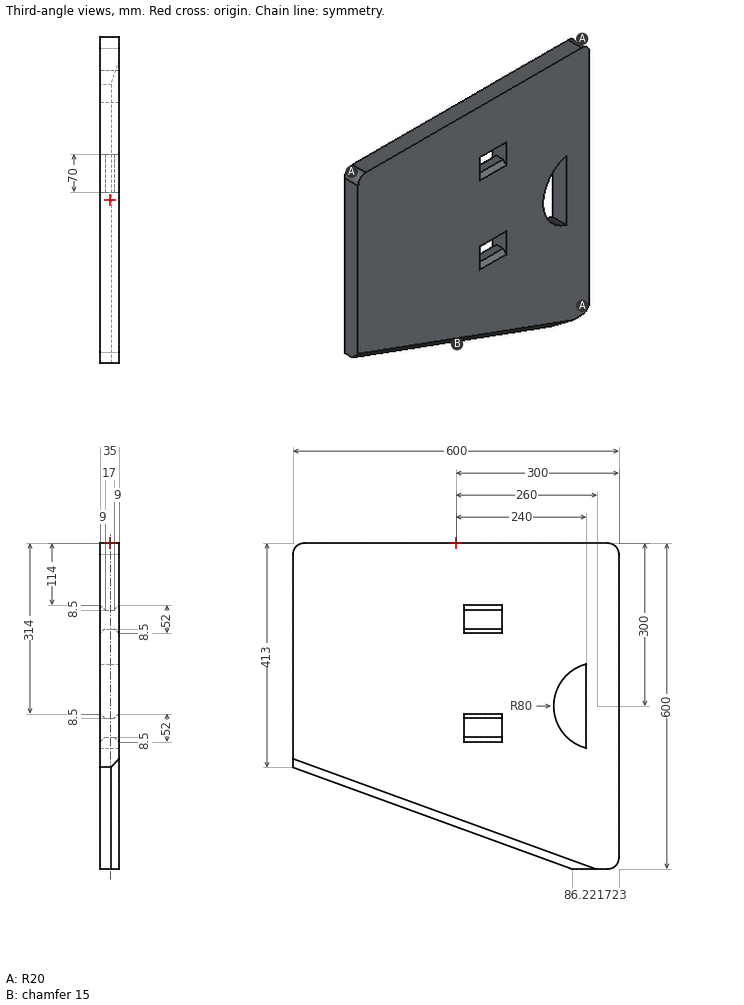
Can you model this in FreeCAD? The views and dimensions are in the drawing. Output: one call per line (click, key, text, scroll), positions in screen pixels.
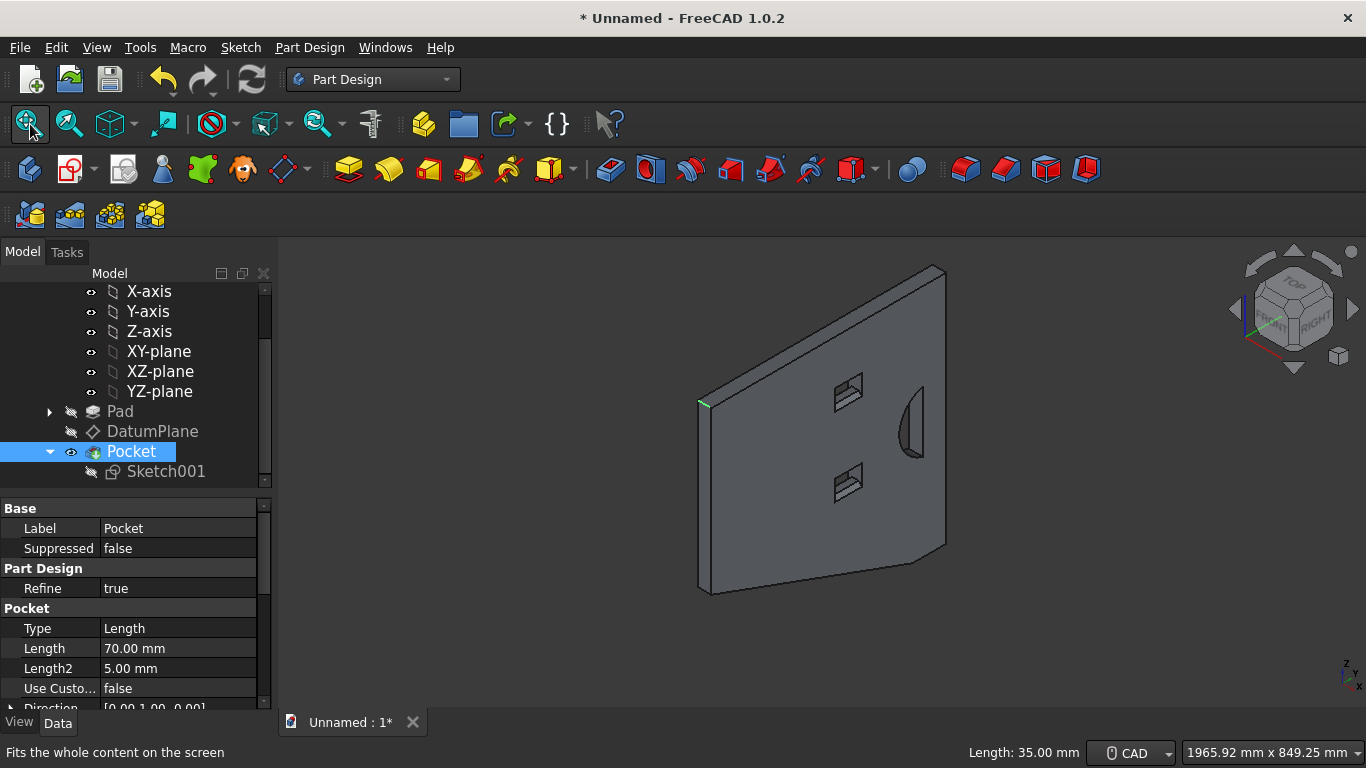
key(2)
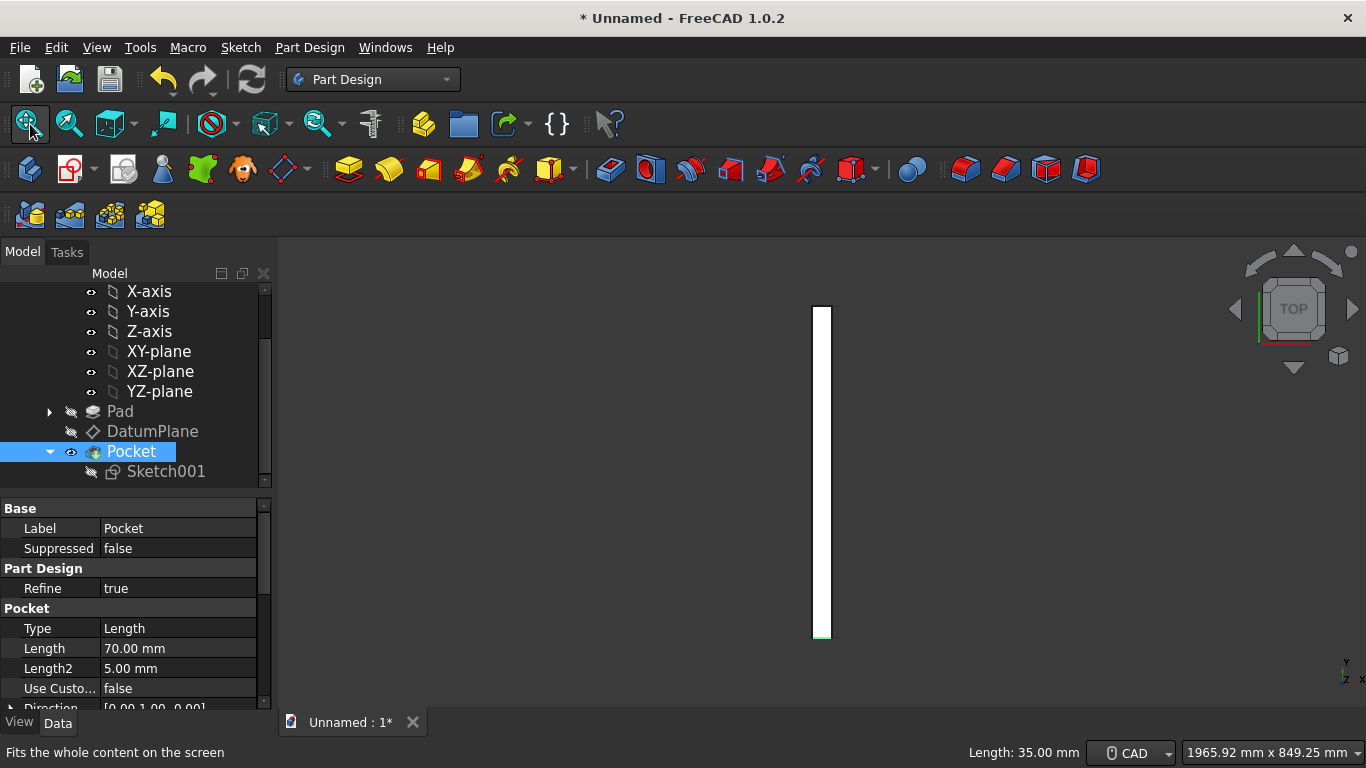
scroll(822, 305, up, 4)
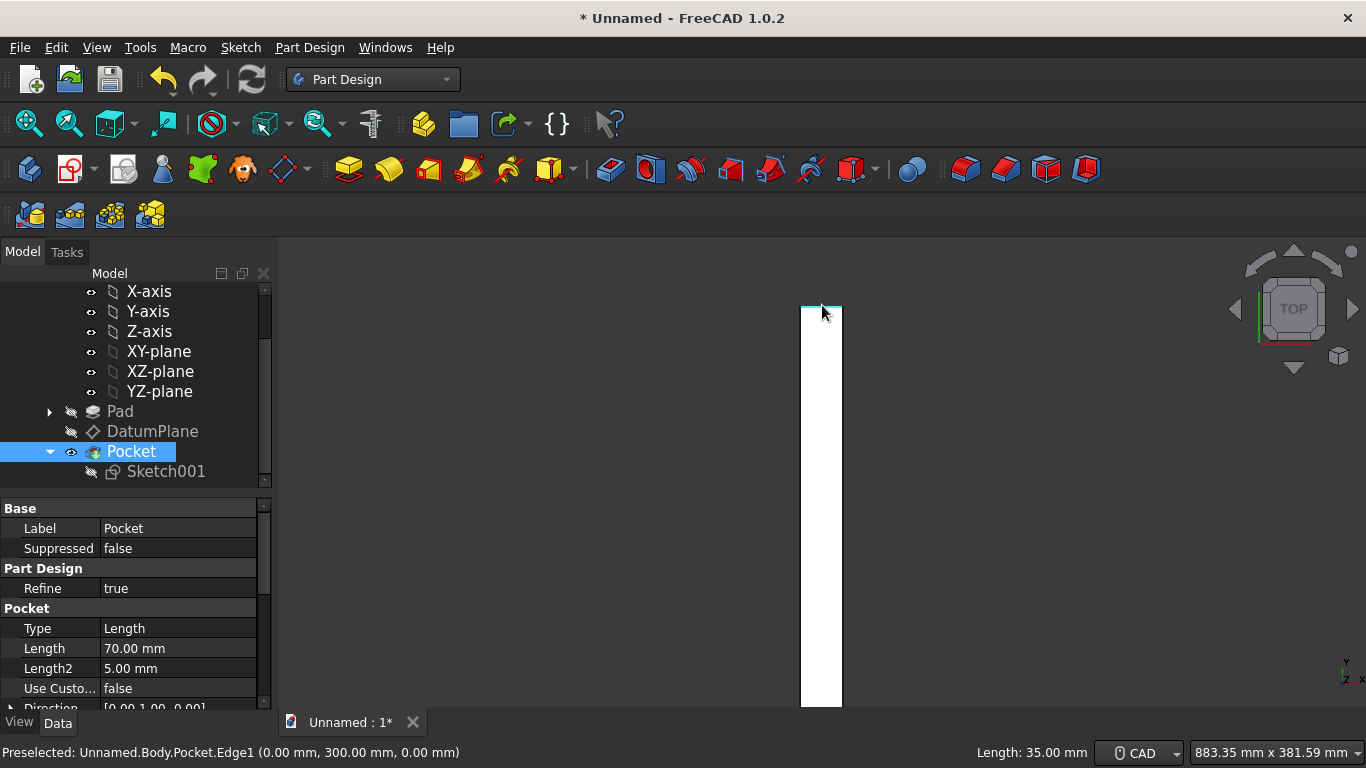
click(30, 124)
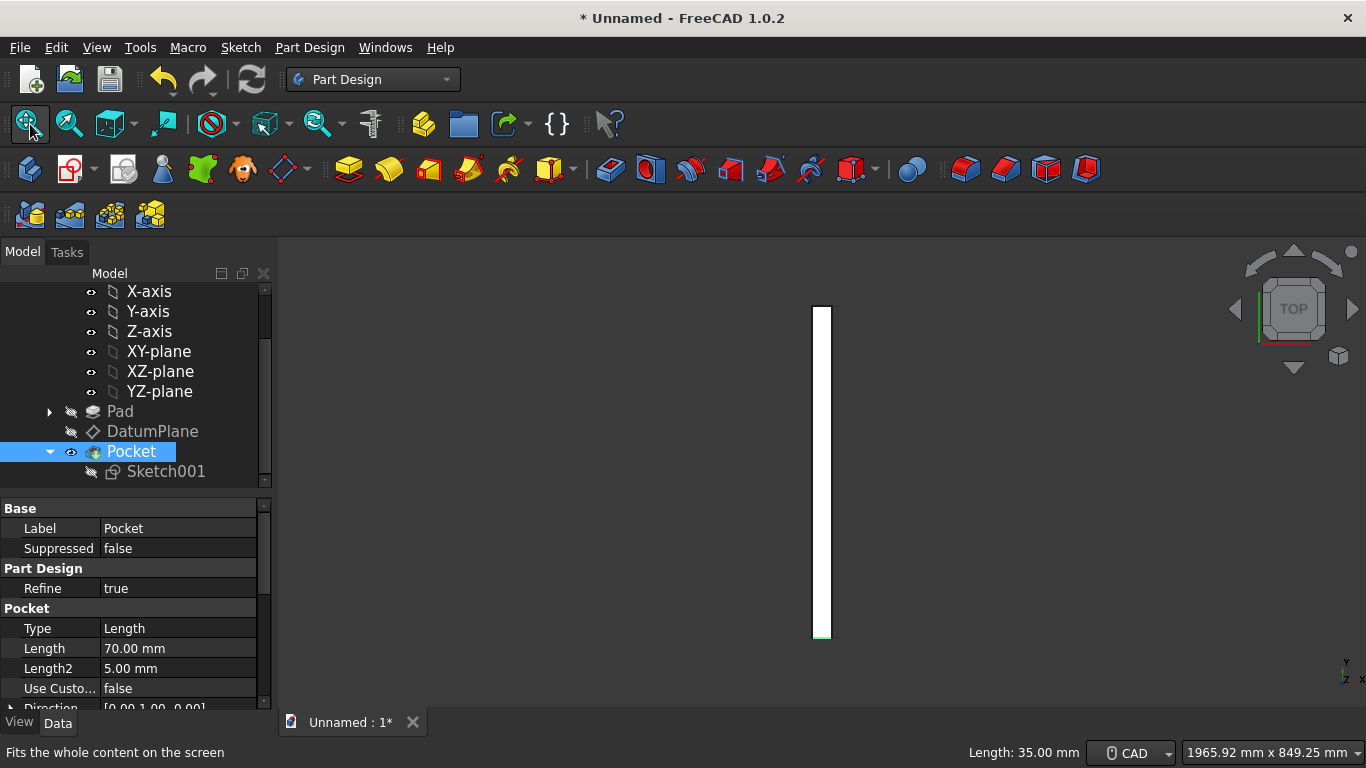
key(1)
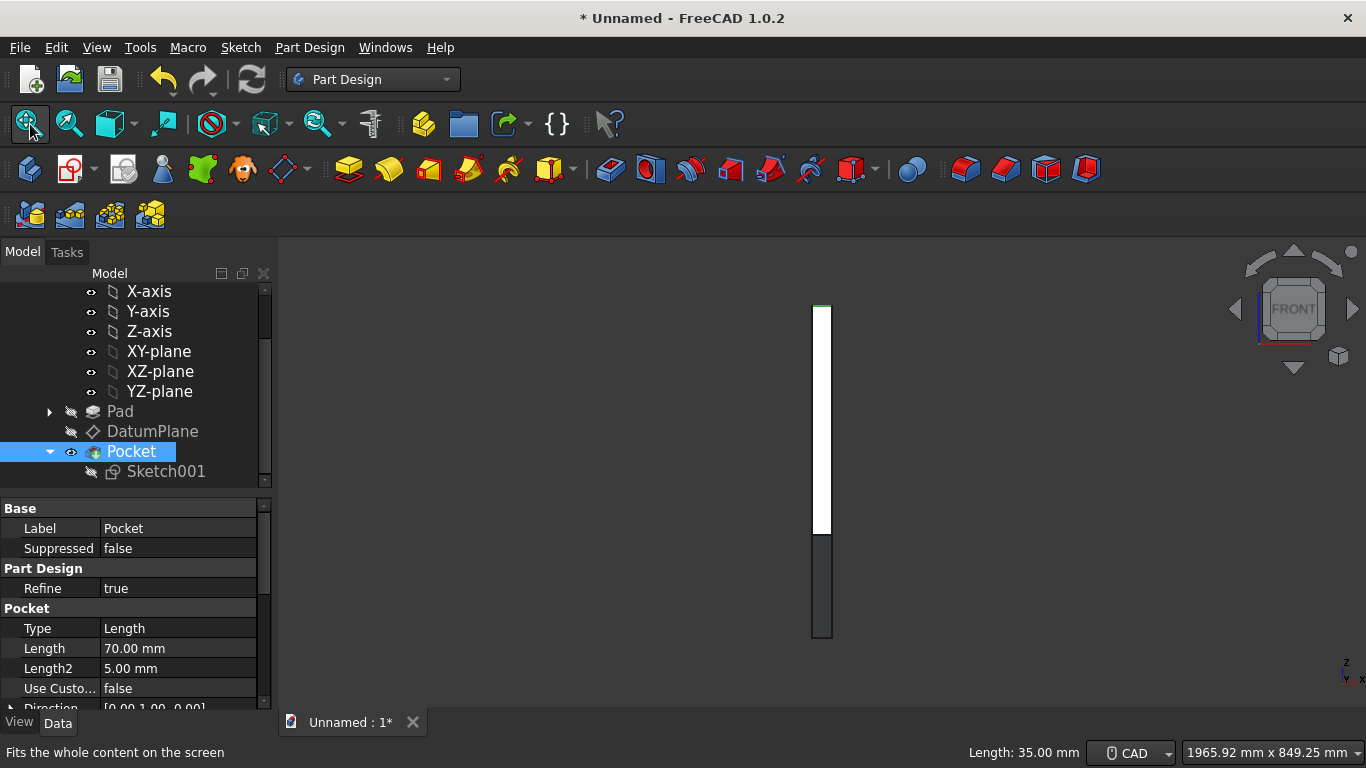
scroll(822, 305, up, 4)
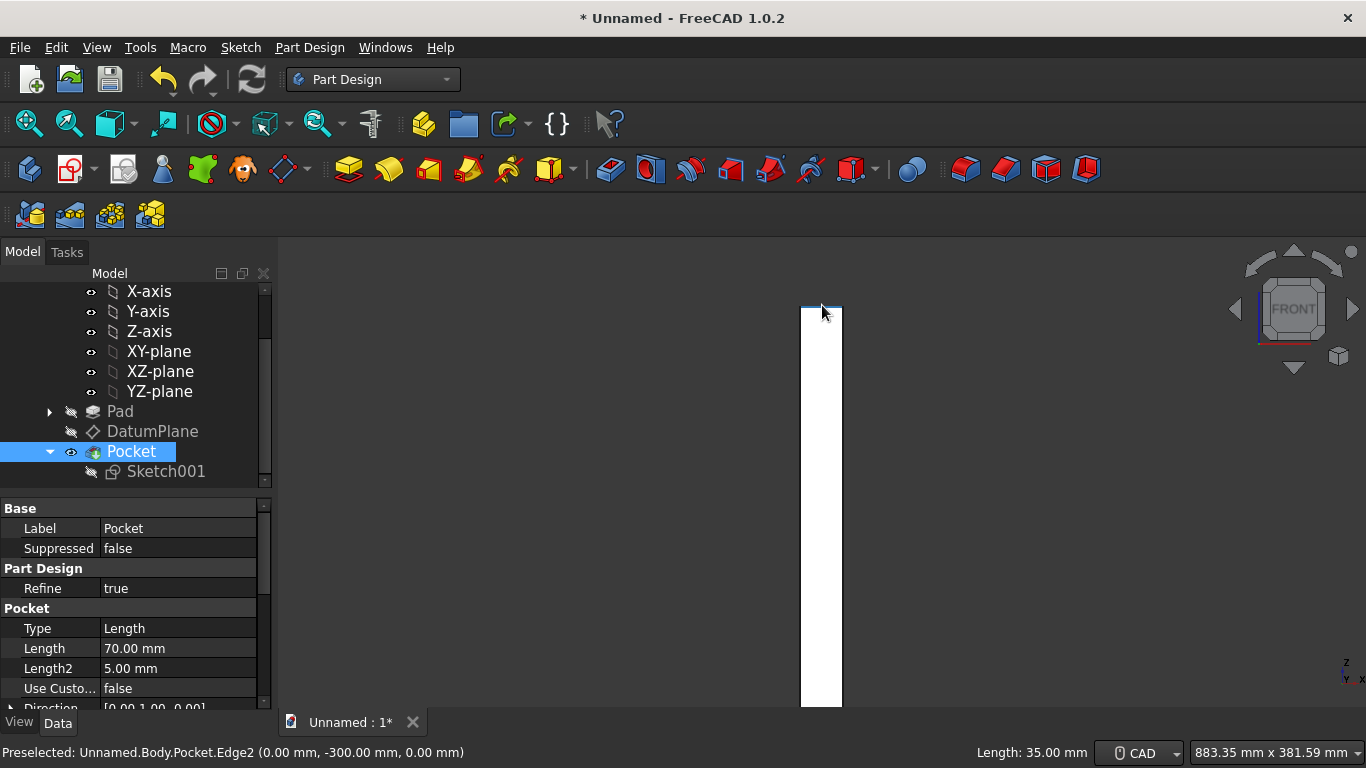
click(30, 124)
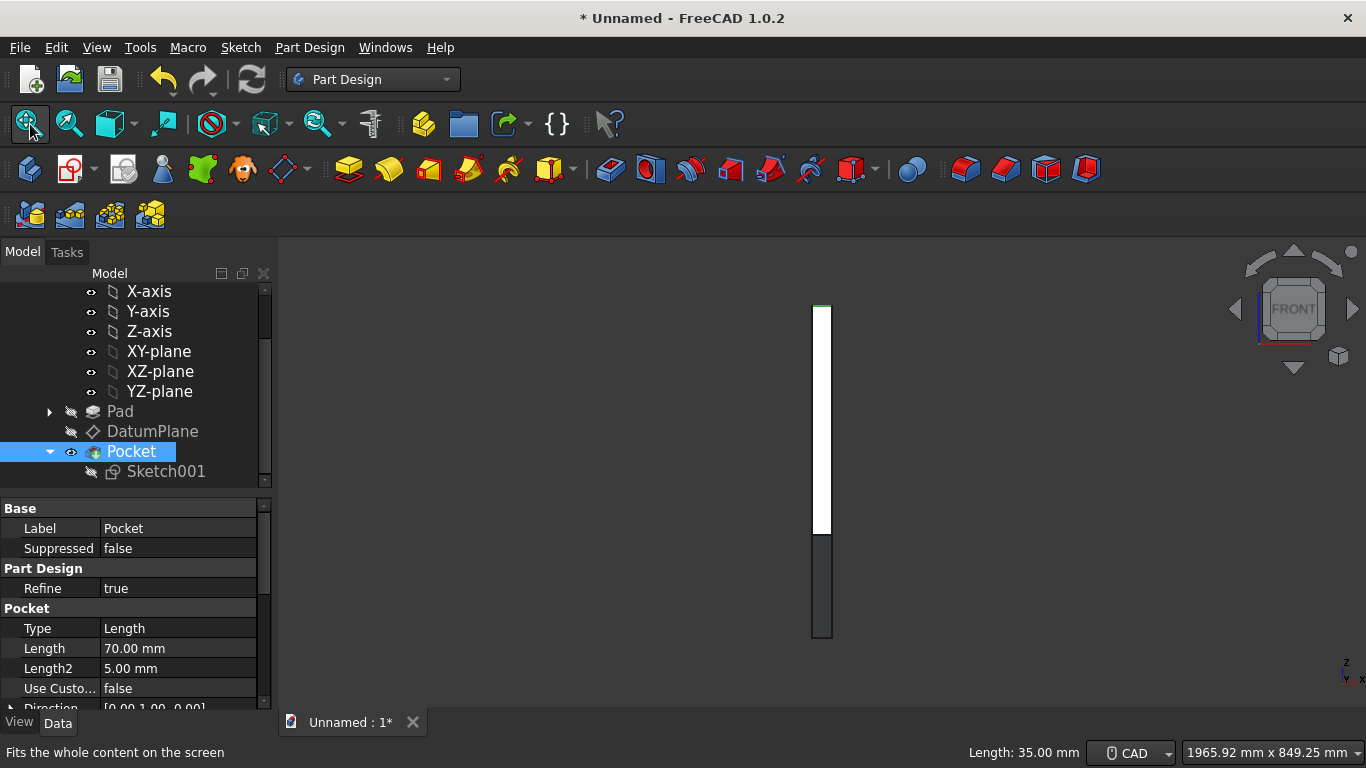
key(3)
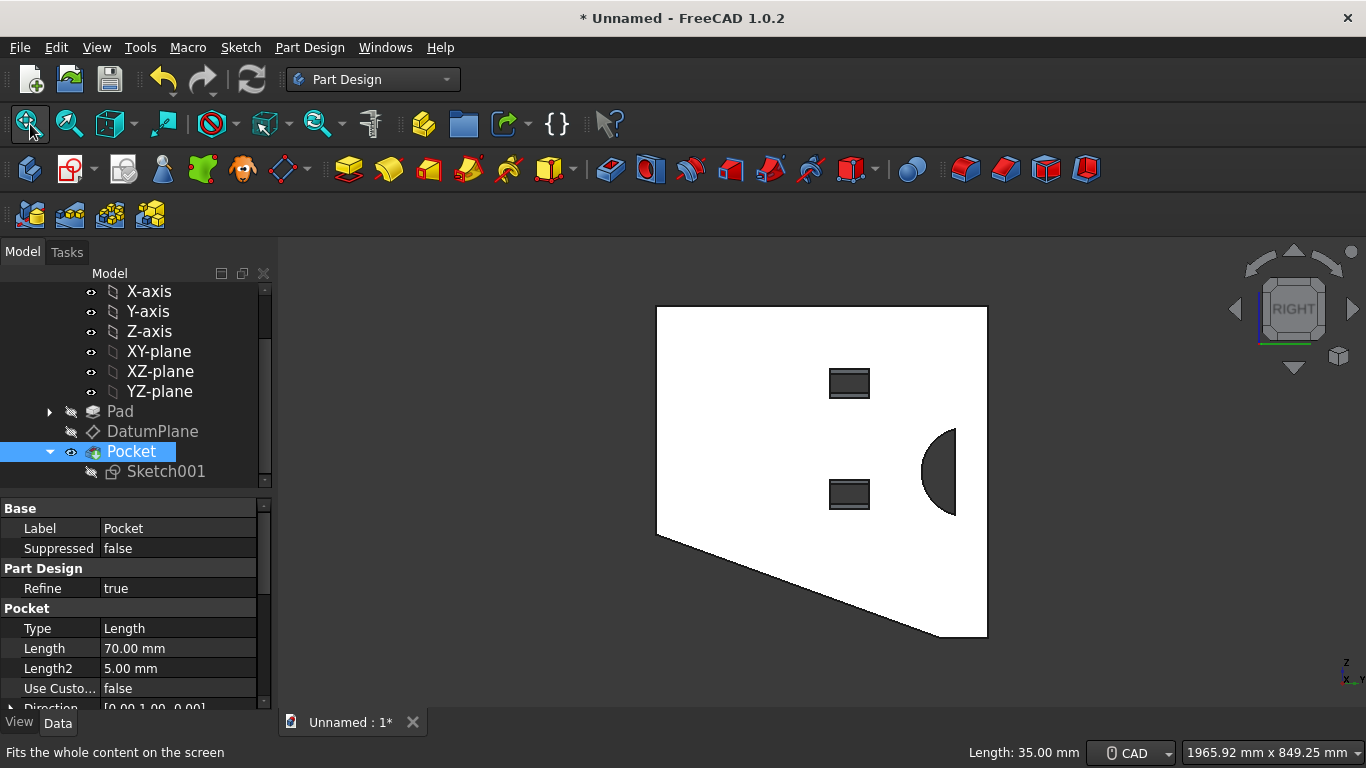
scroll(988, 305, up, 4)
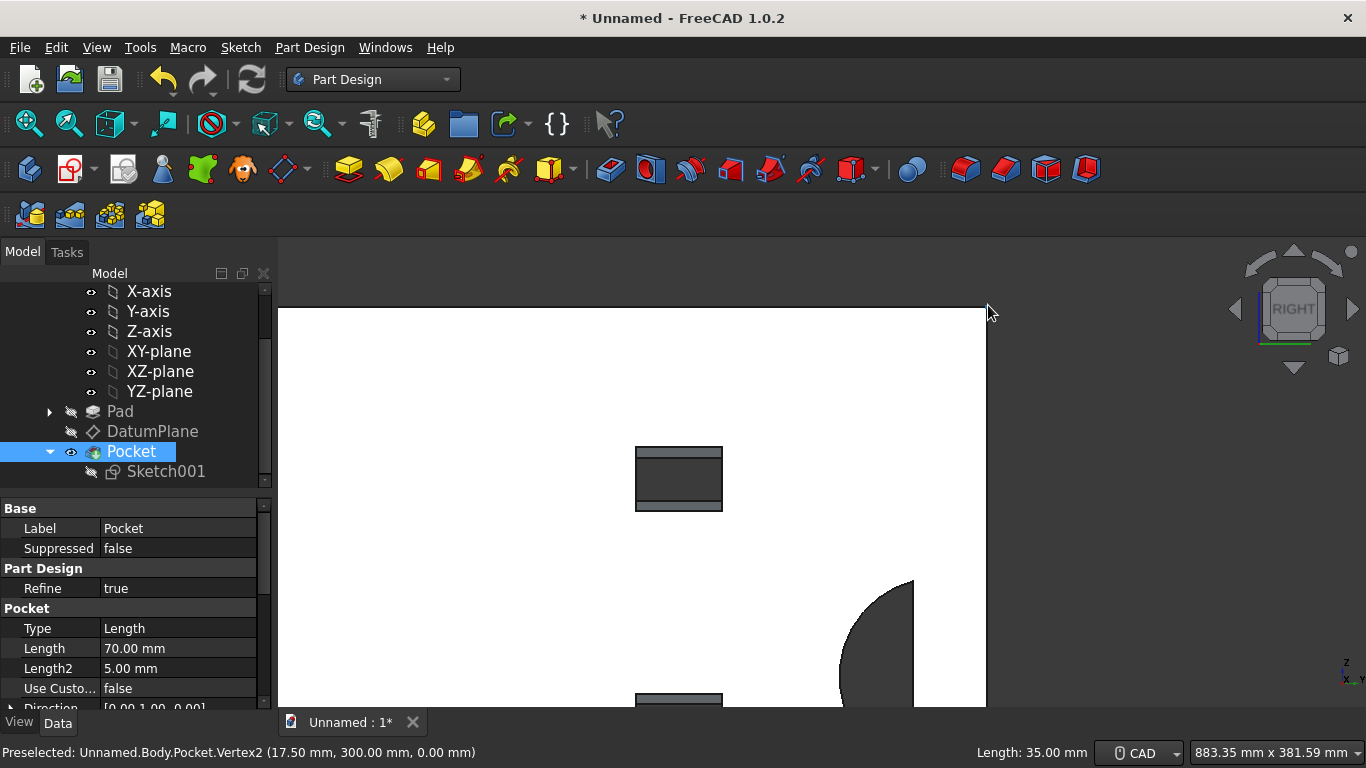
click(30, 124)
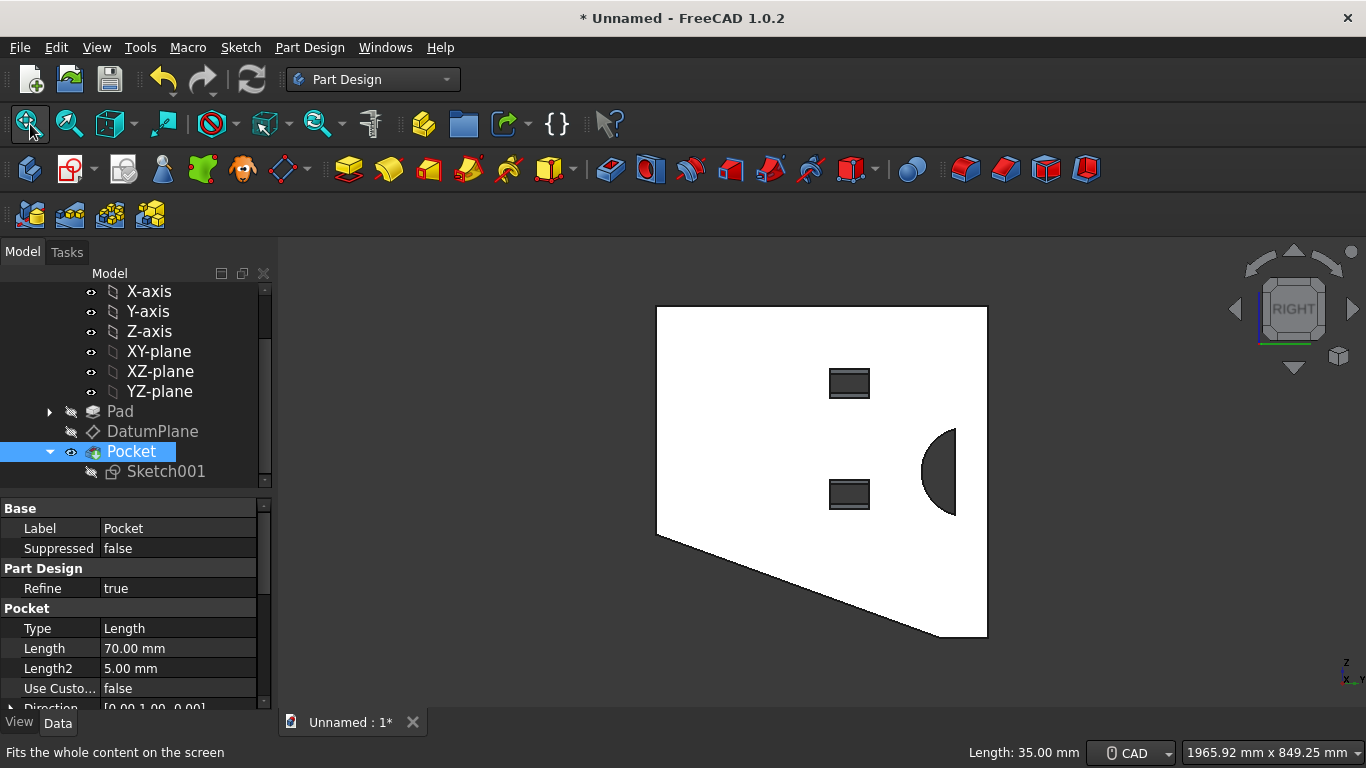
key(5)